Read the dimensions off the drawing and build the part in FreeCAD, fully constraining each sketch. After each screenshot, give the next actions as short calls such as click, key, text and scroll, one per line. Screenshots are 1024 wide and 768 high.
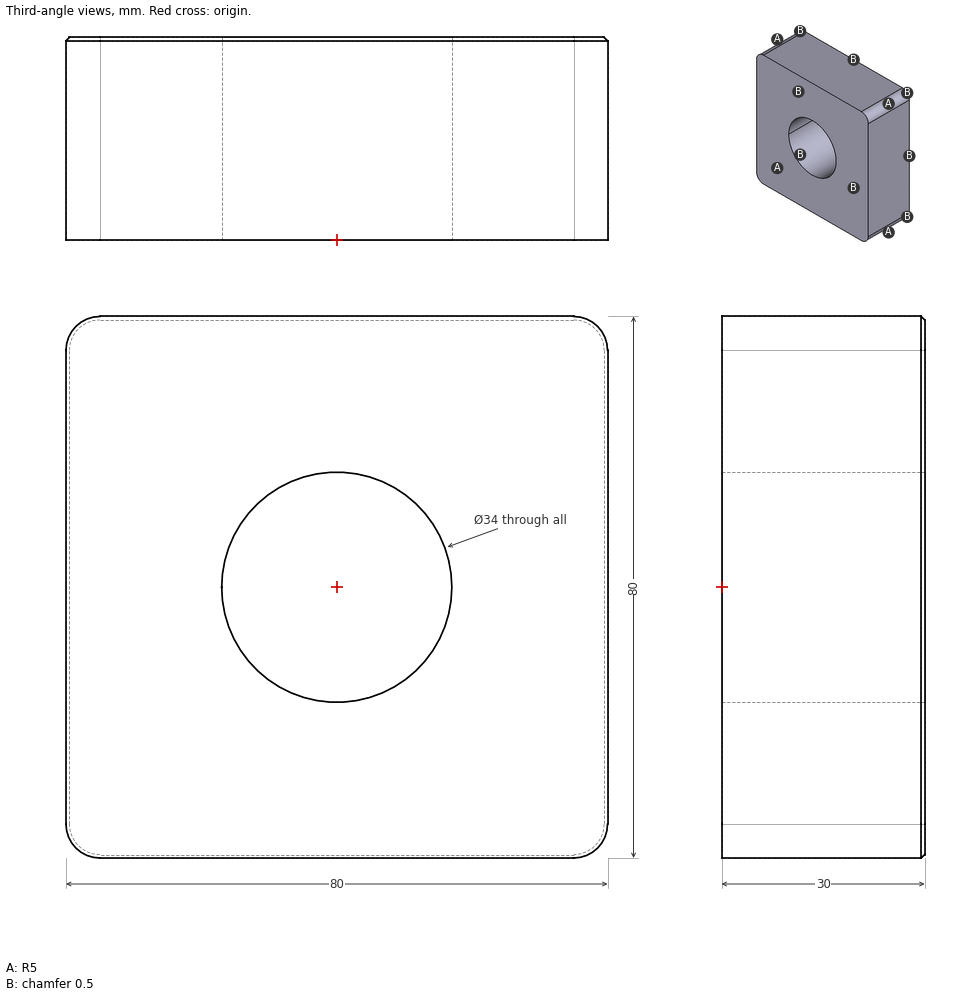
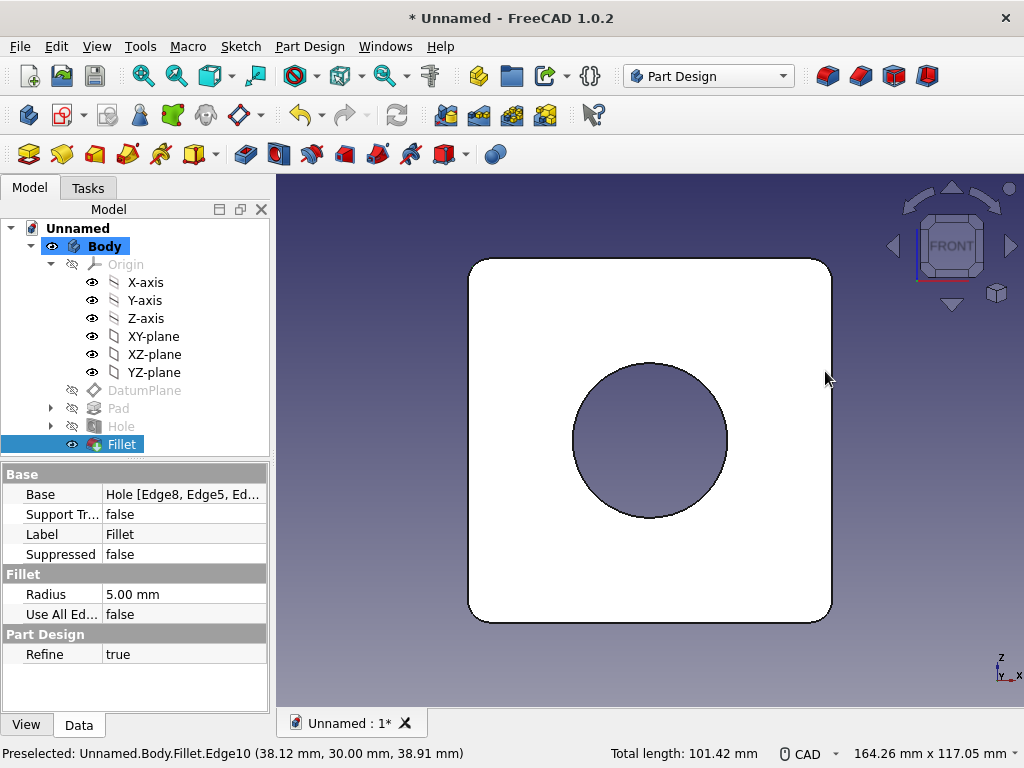
key(3)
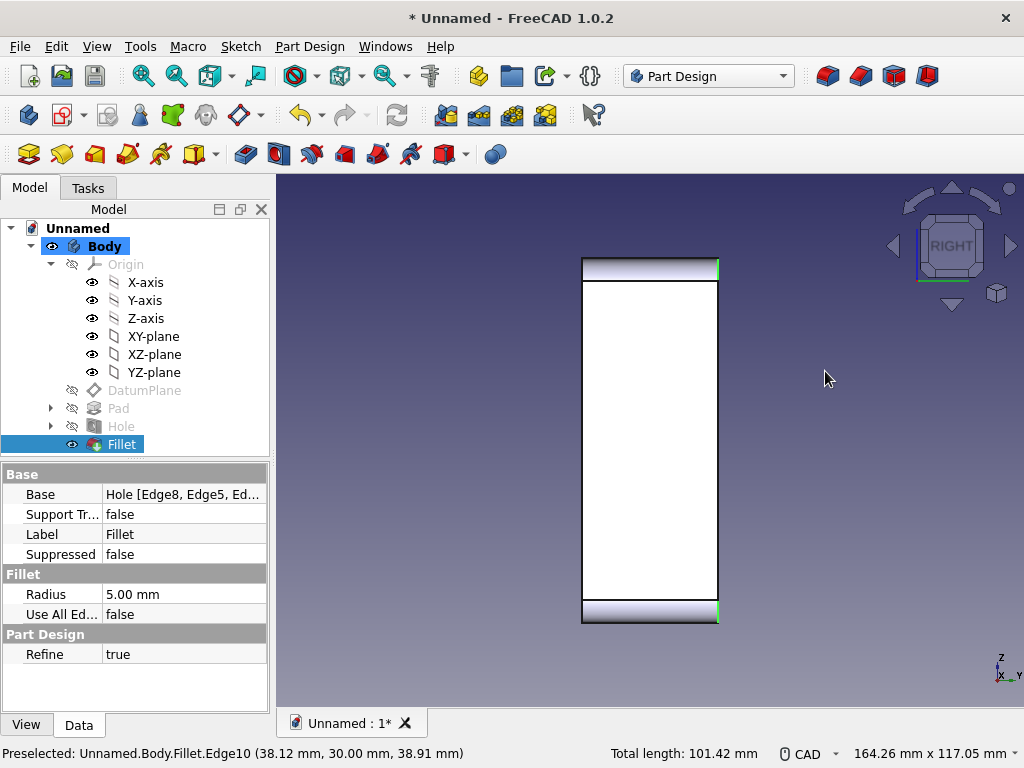
click(718, 440, ctrl)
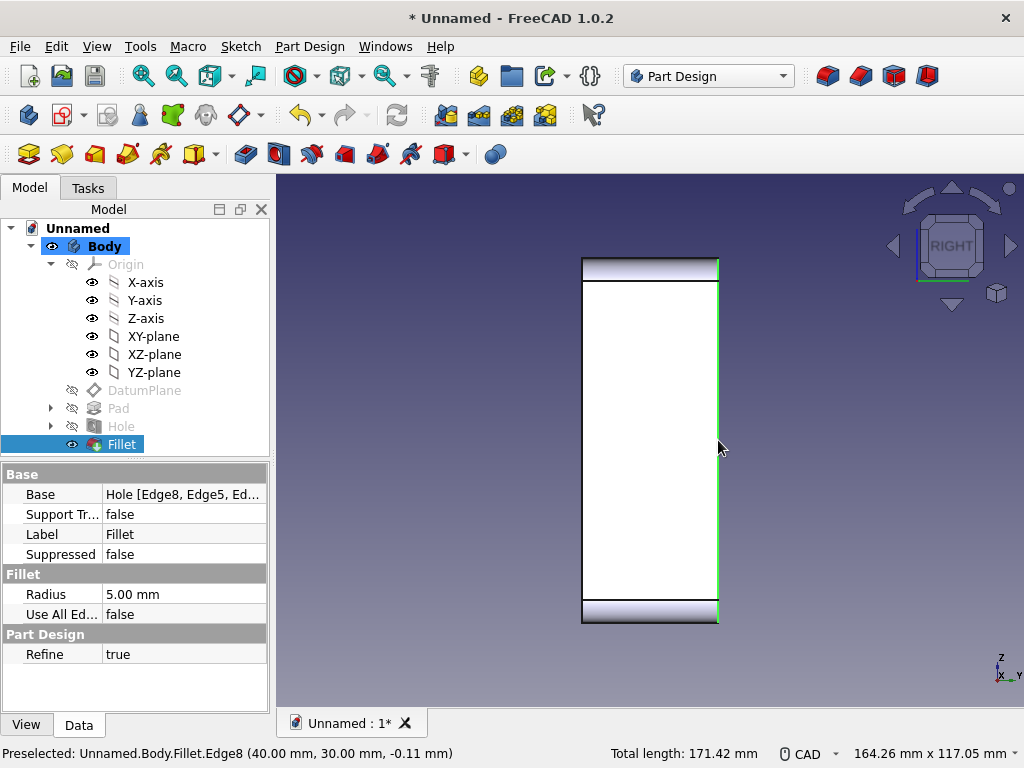
key(5)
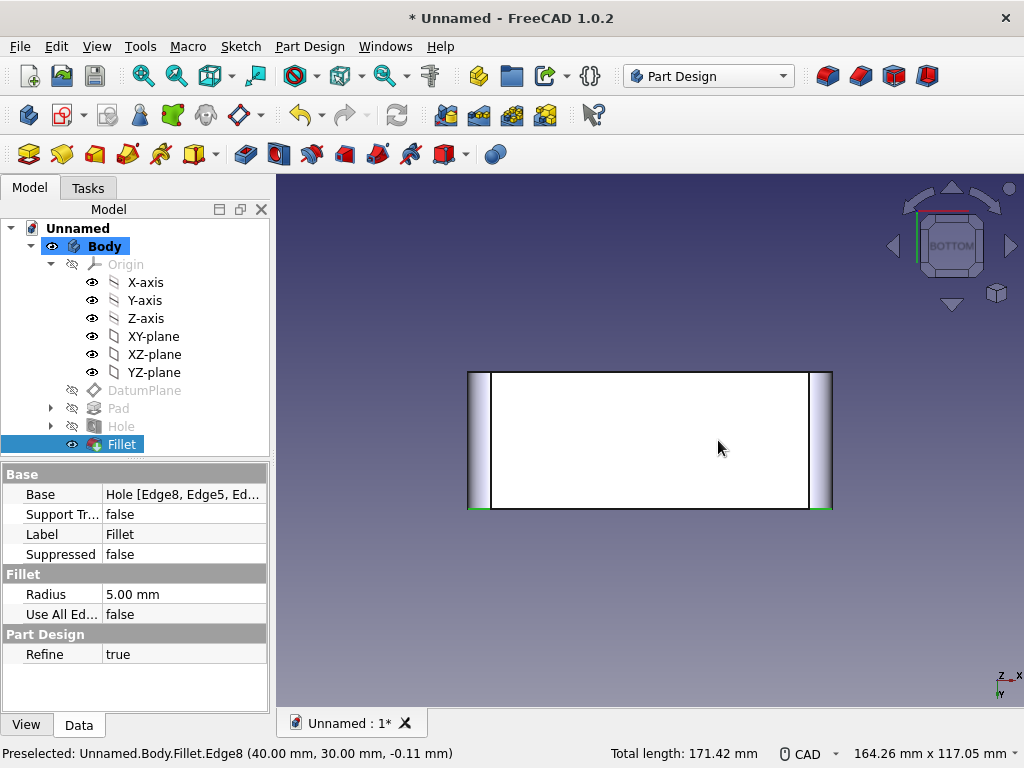
key(4)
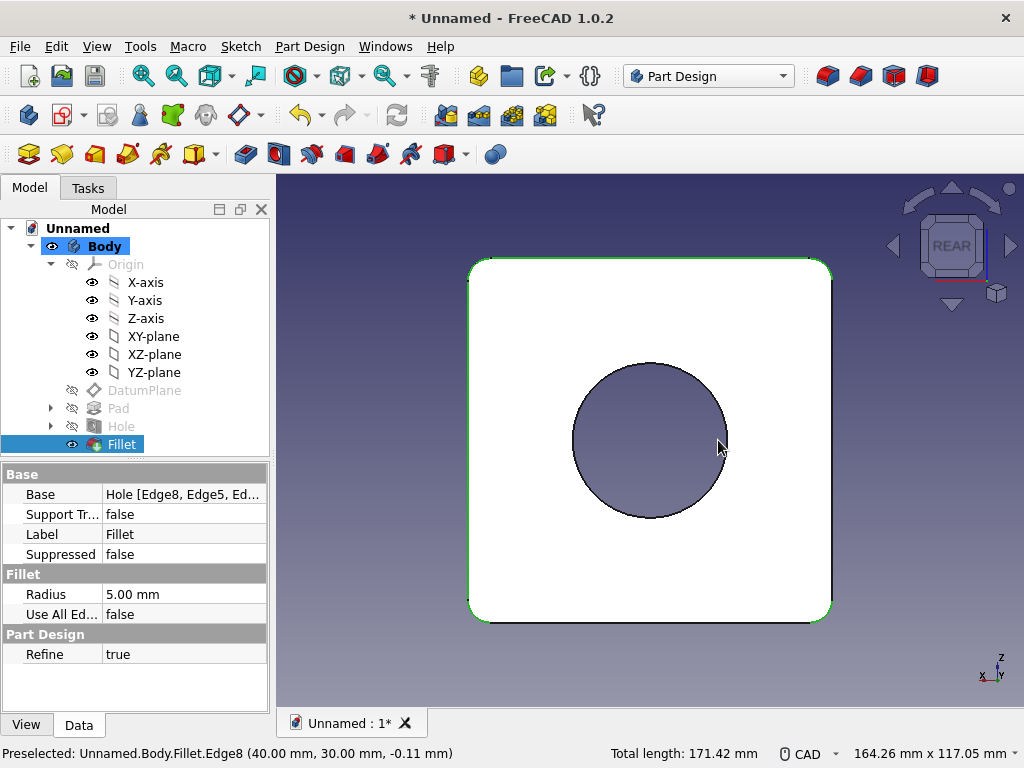
click(832, 440, ctrl)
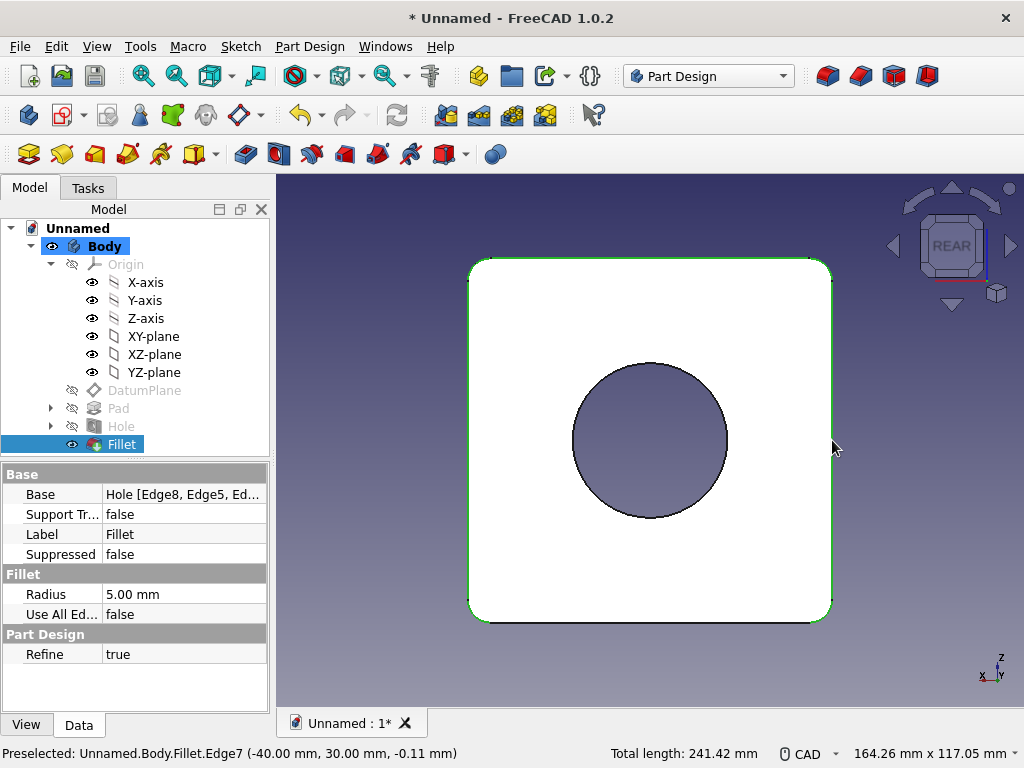
click(650, 622, ctrl)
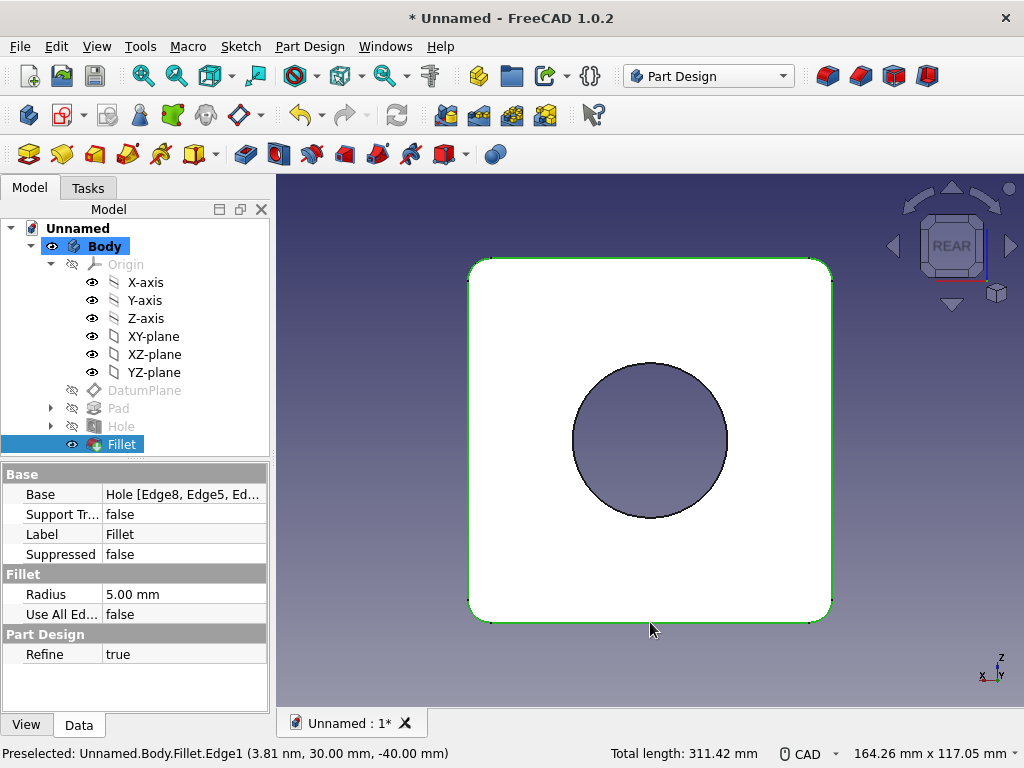
click(861, 76)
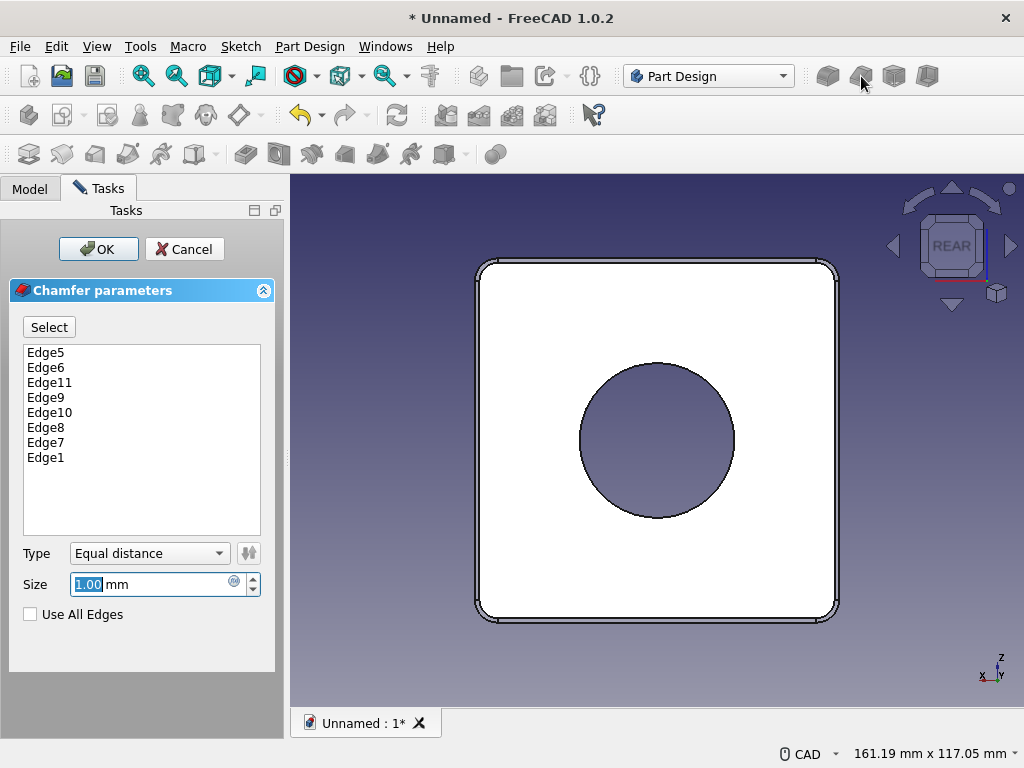
text(0.5)
key(Tab)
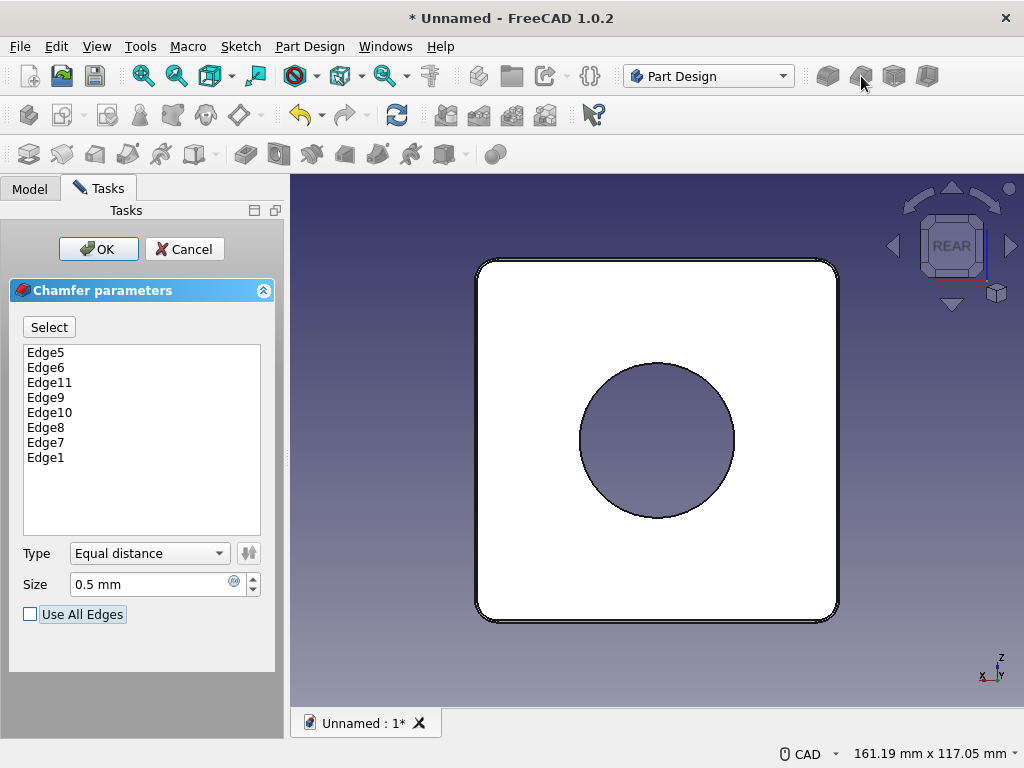
click(99, 249)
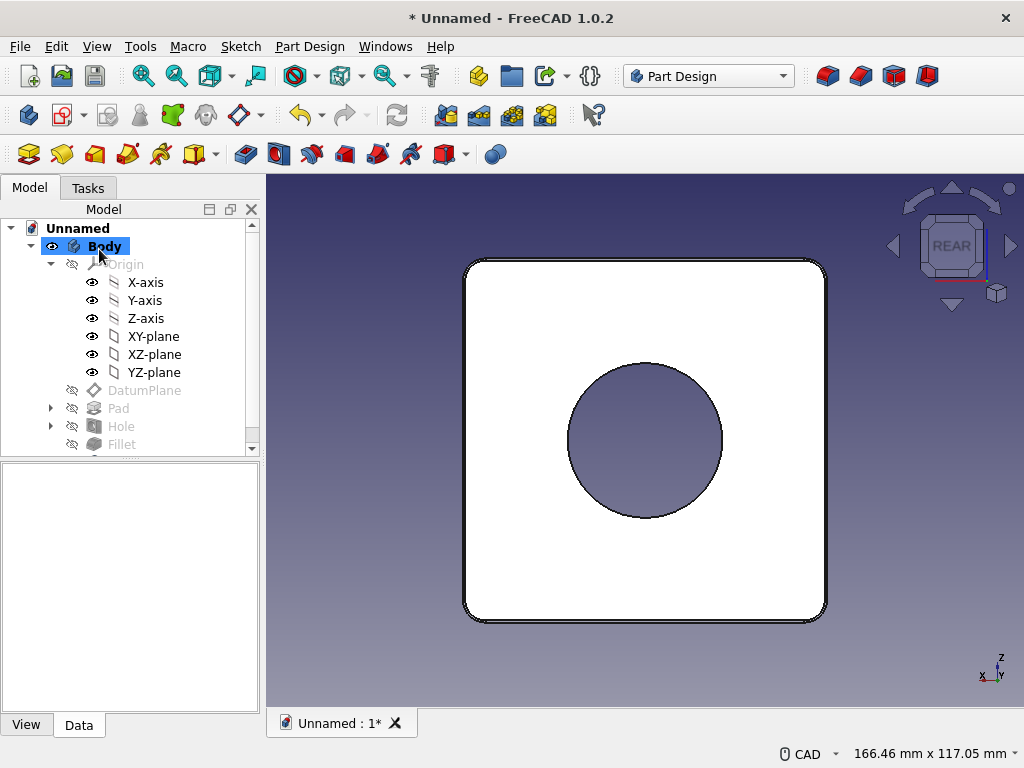
key(0)